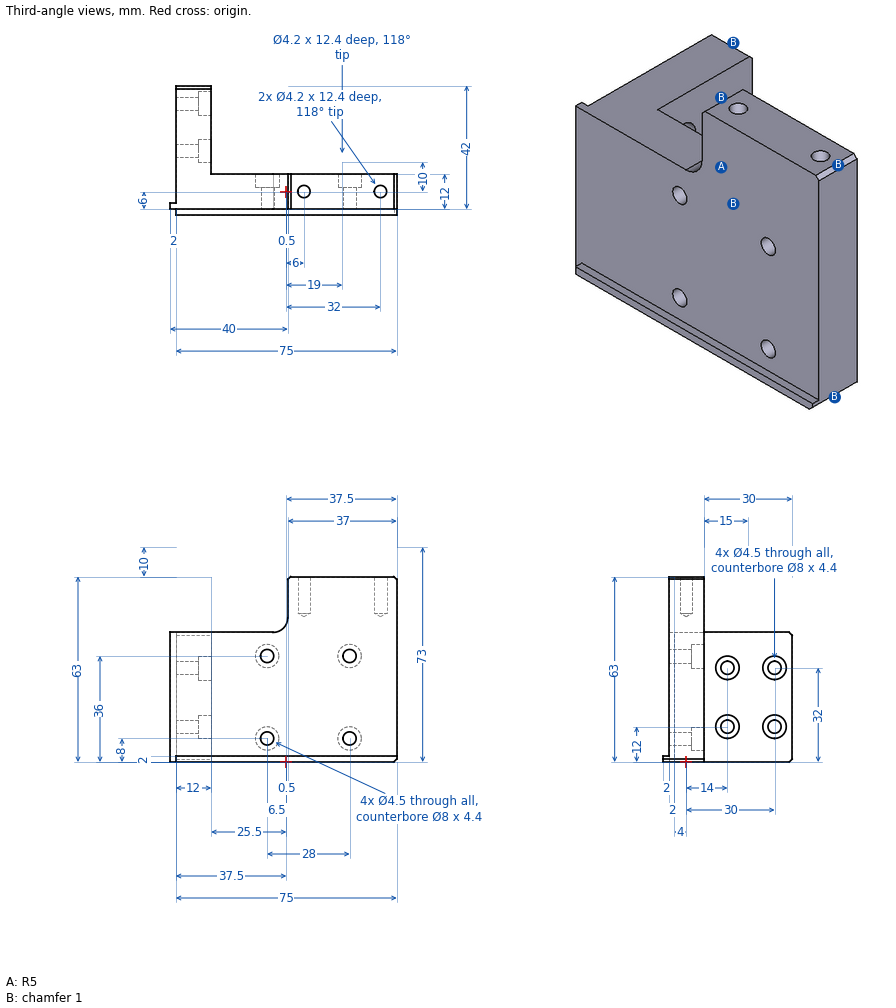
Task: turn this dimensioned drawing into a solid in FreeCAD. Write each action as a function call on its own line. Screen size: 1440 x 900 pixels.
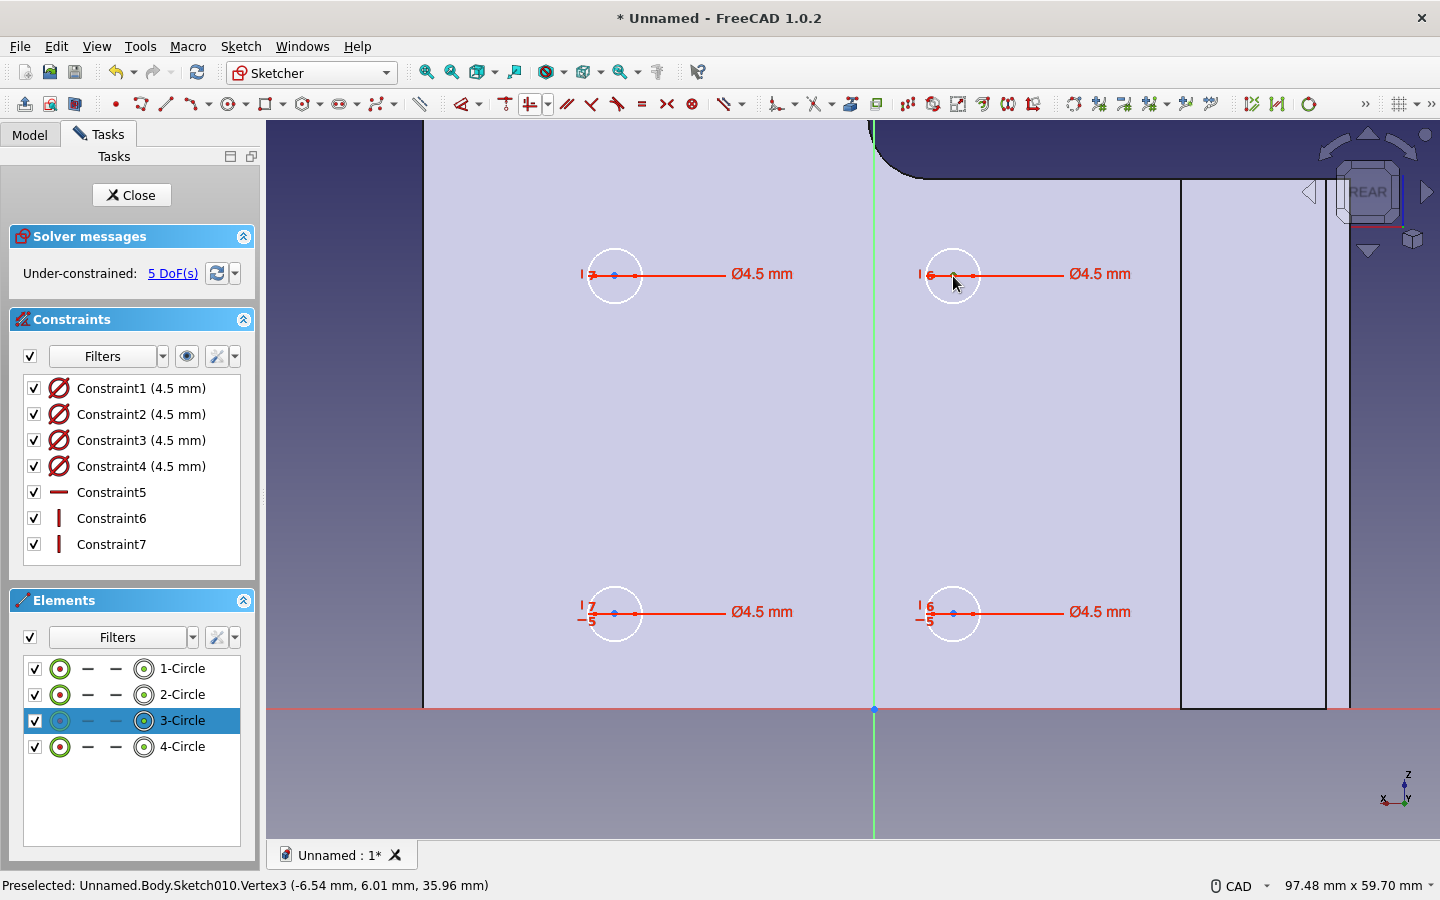
click(615, 276)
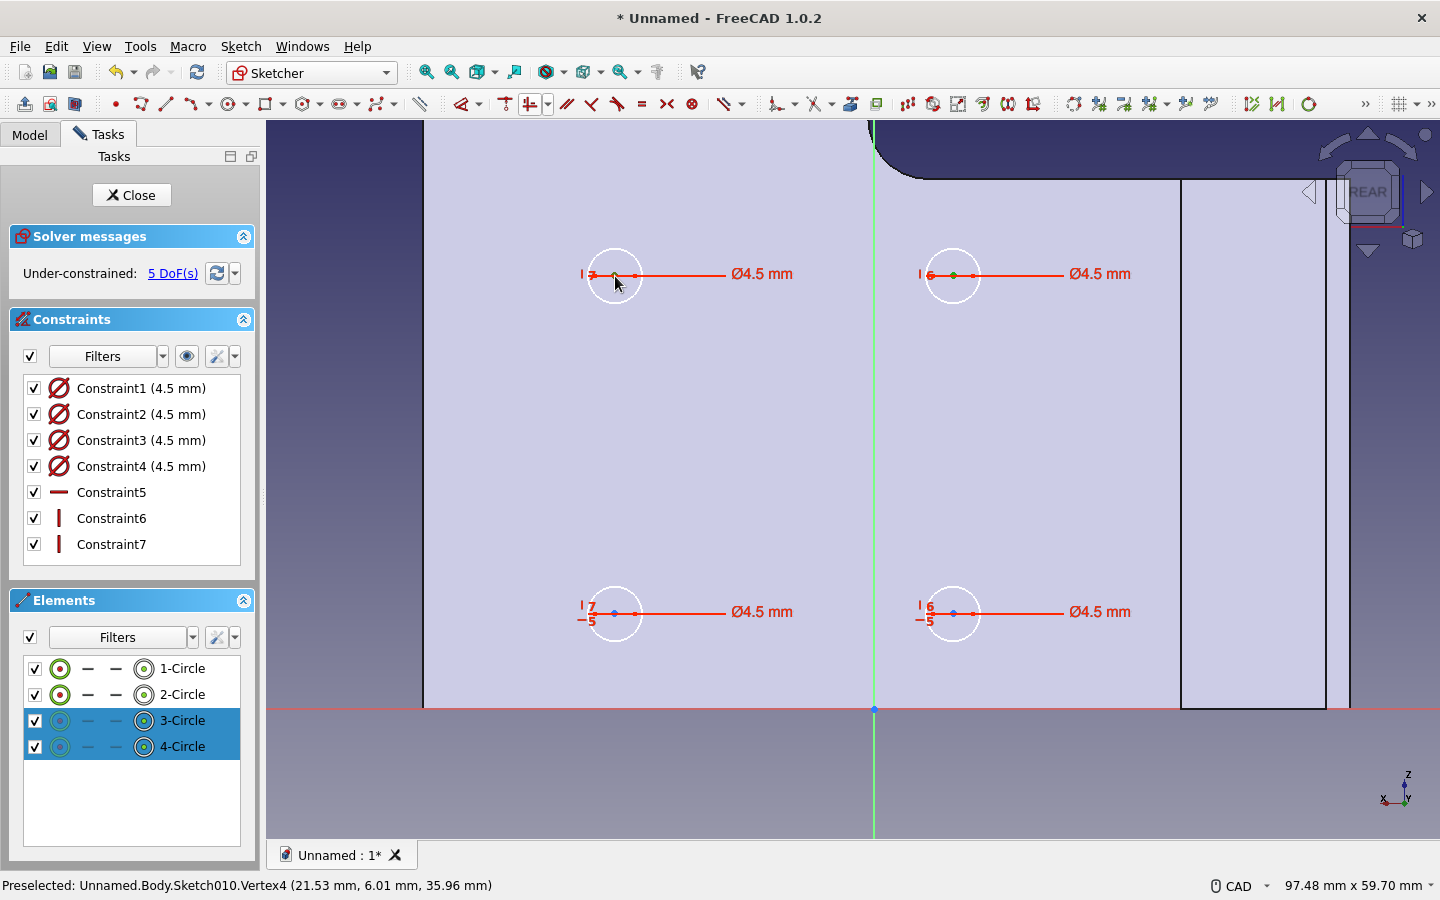
key(h)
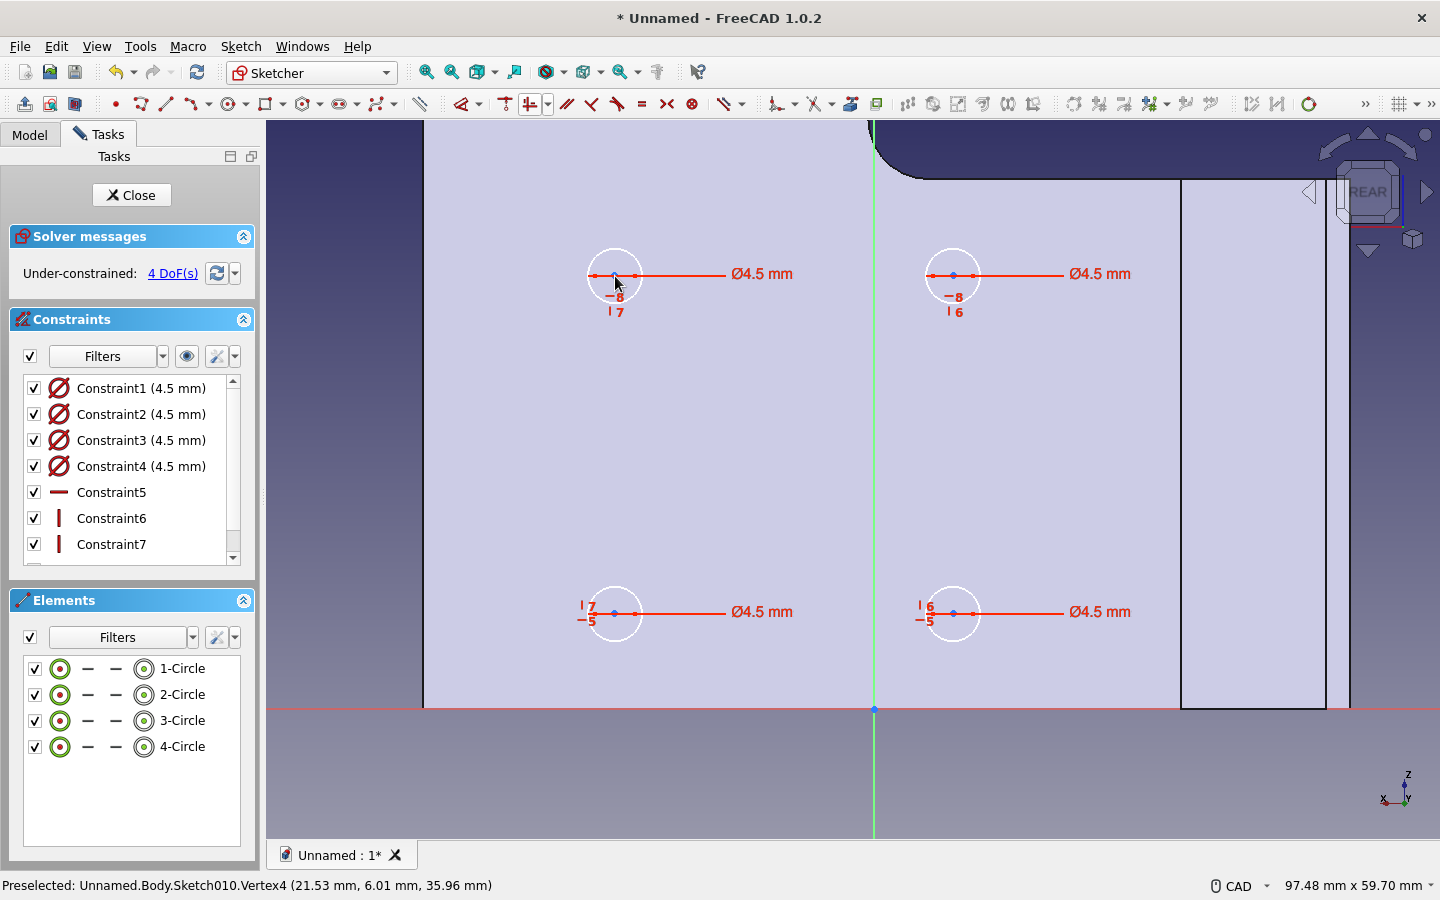
click(460, 104)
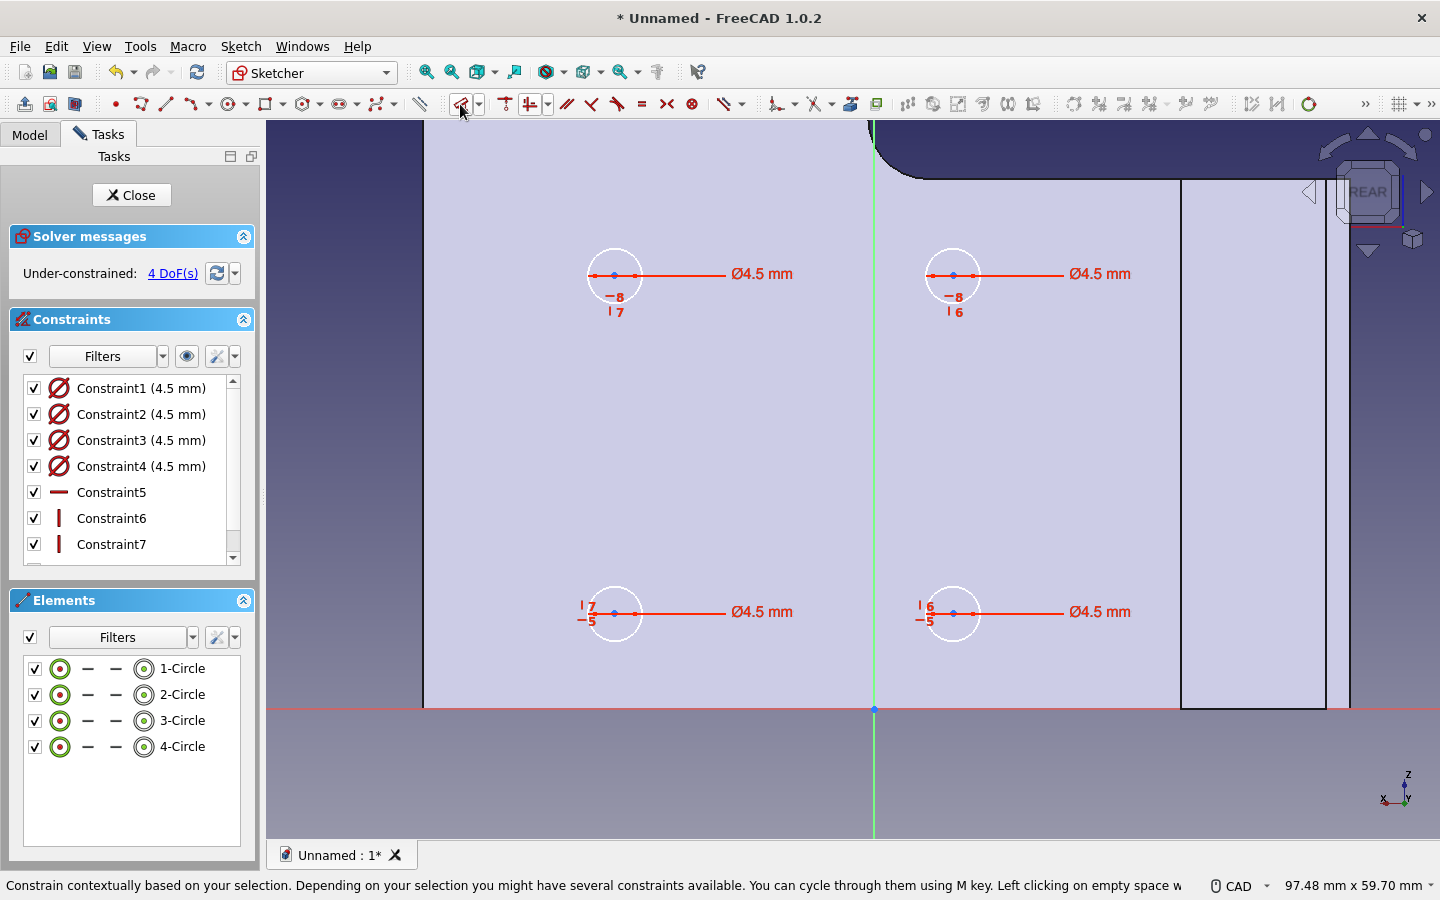
click(953, 614)
click(987, 662)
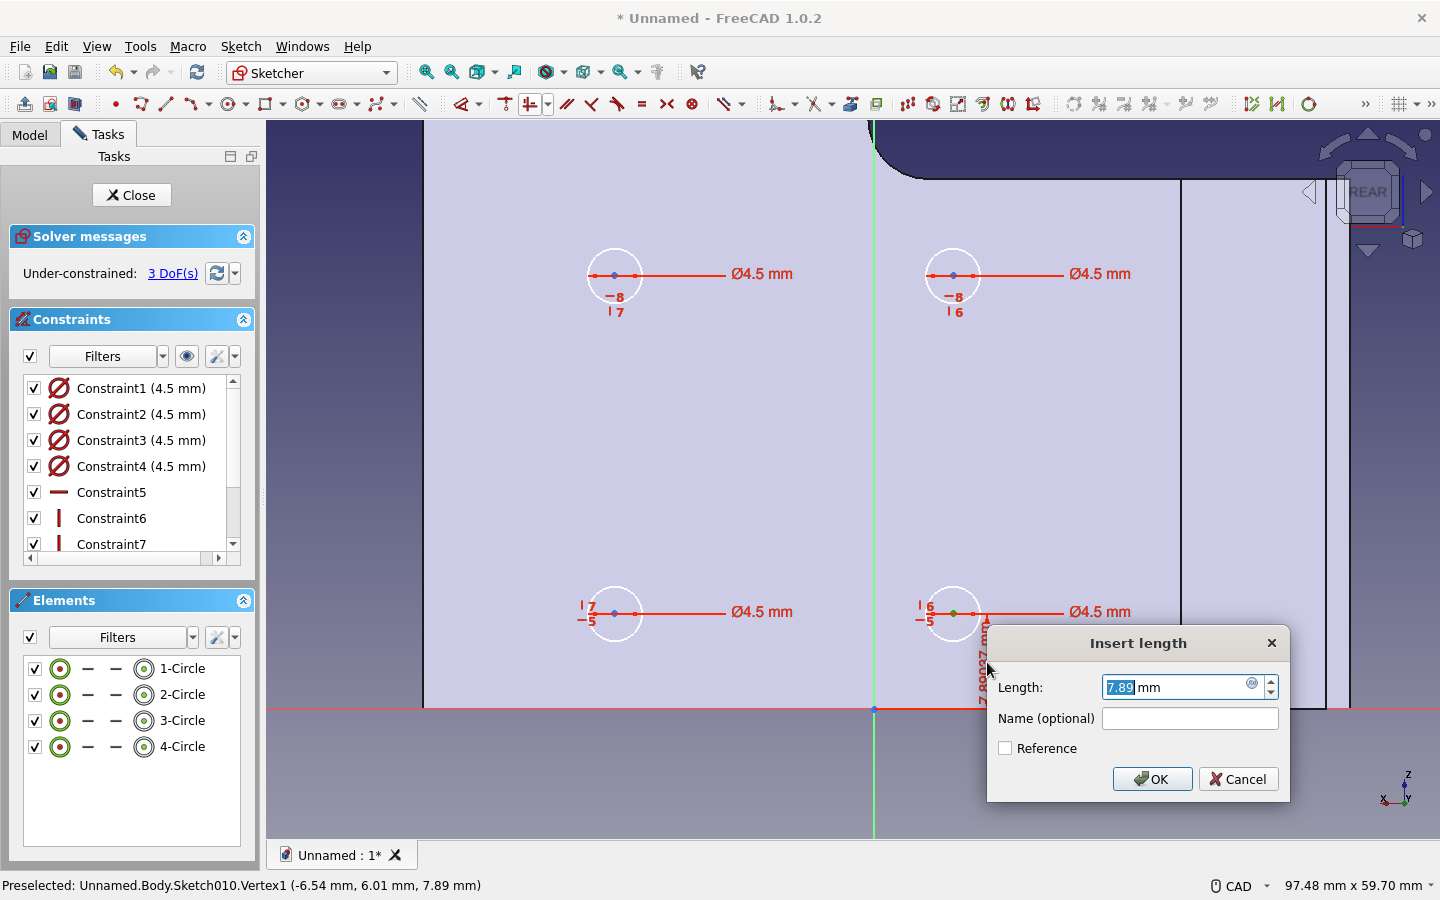
text(8)
key(Return)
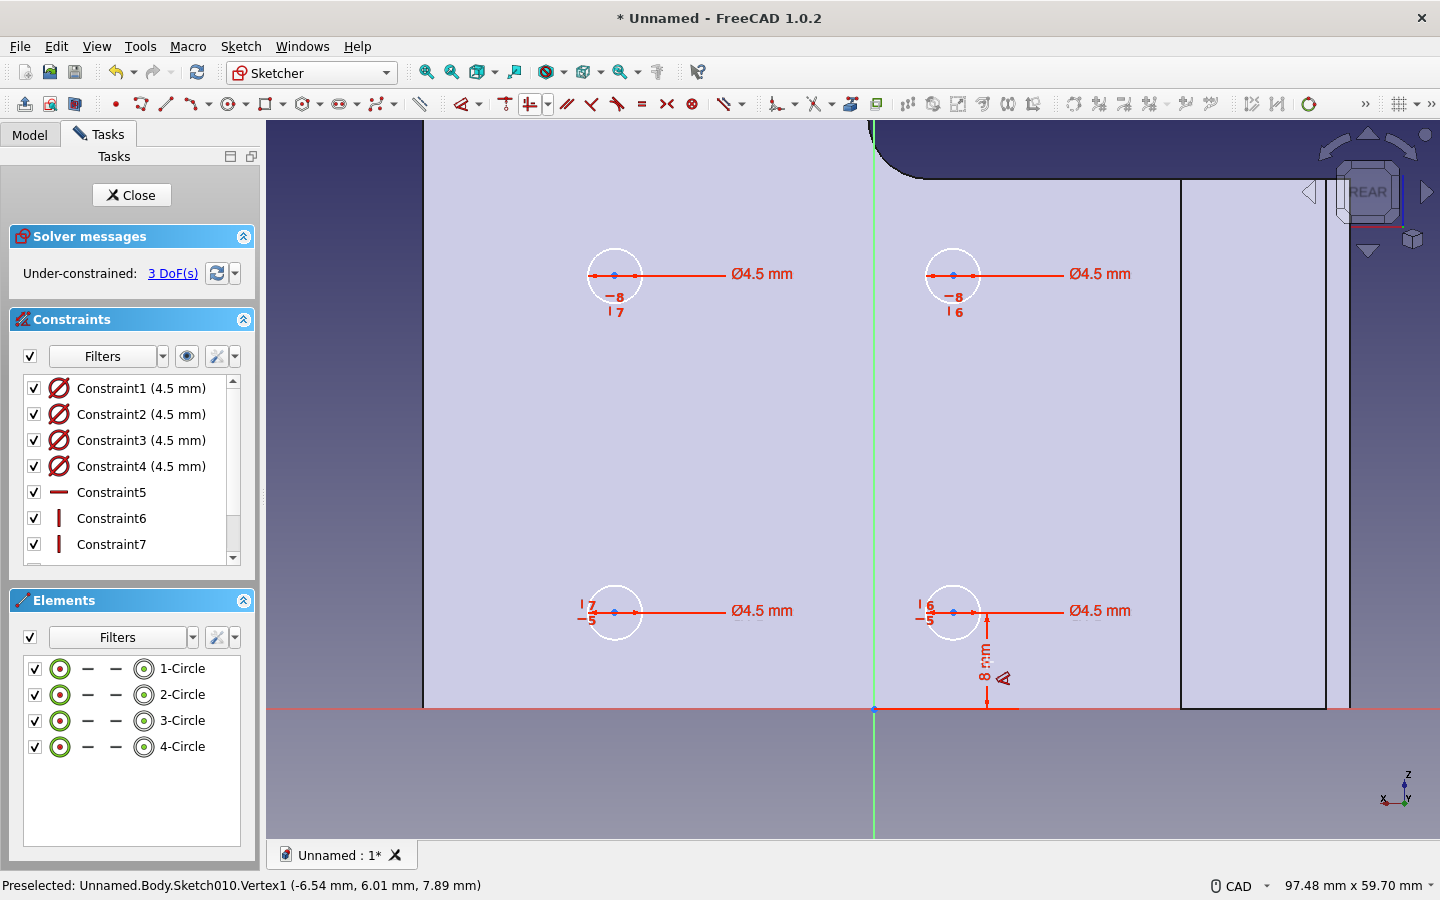
click(953, 276)
click(987, 493)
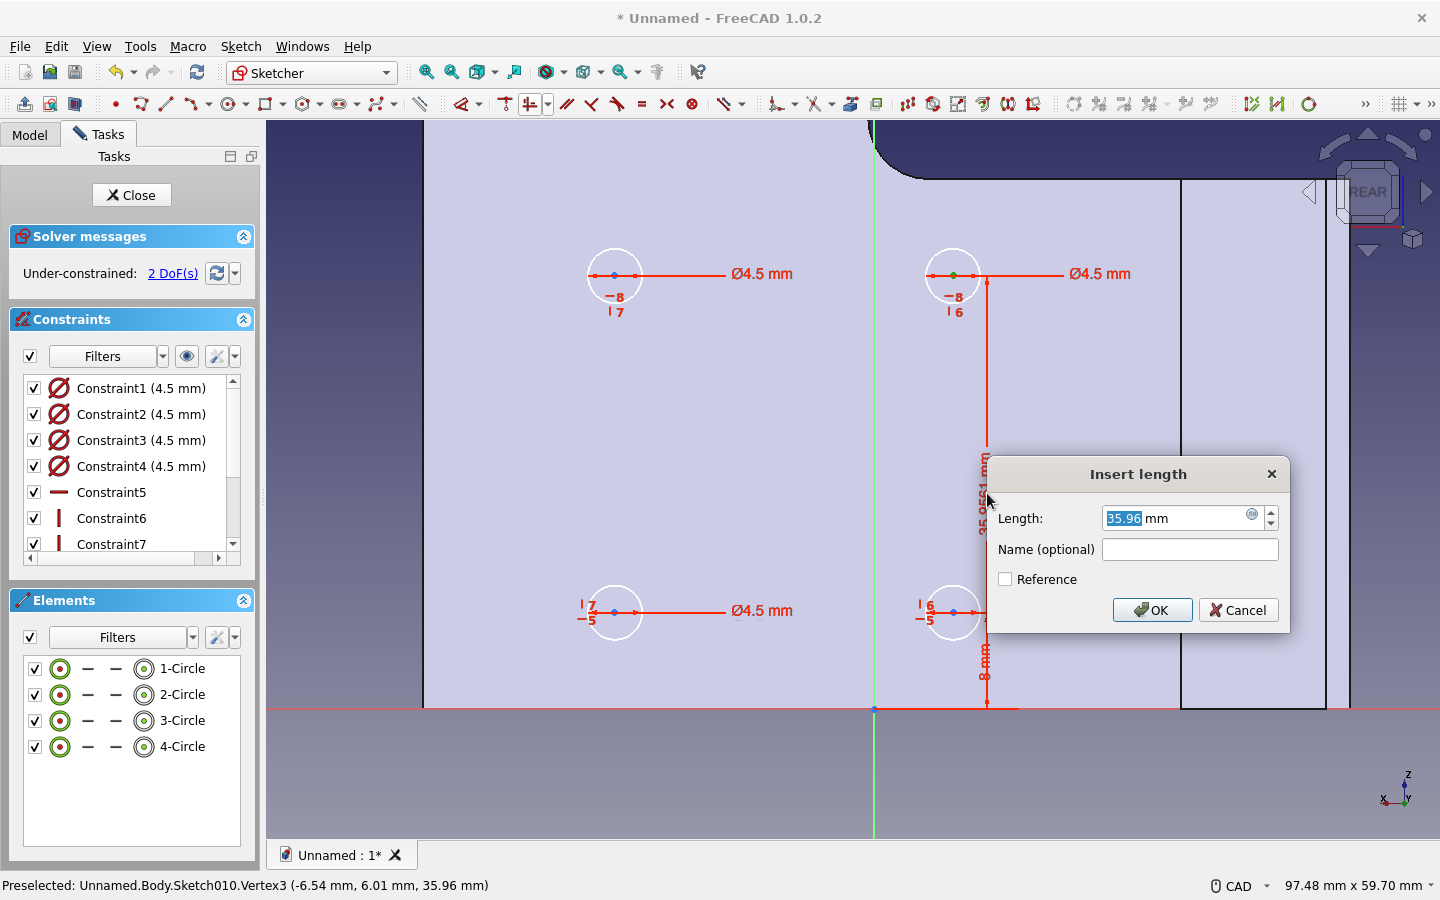
text(36)
key(Return)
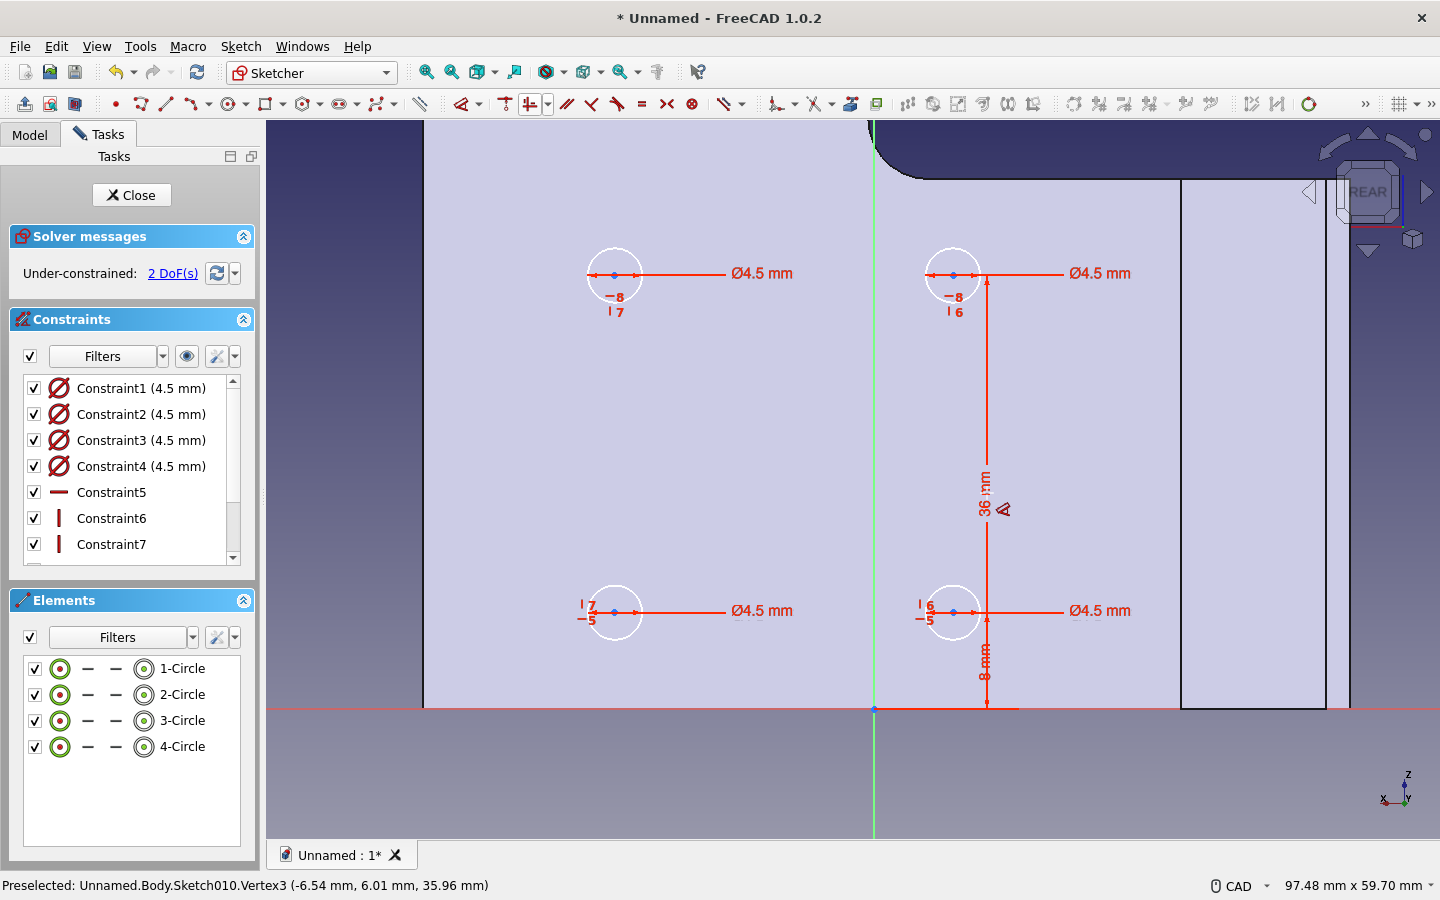
click(953, 613)
click(914, 743)